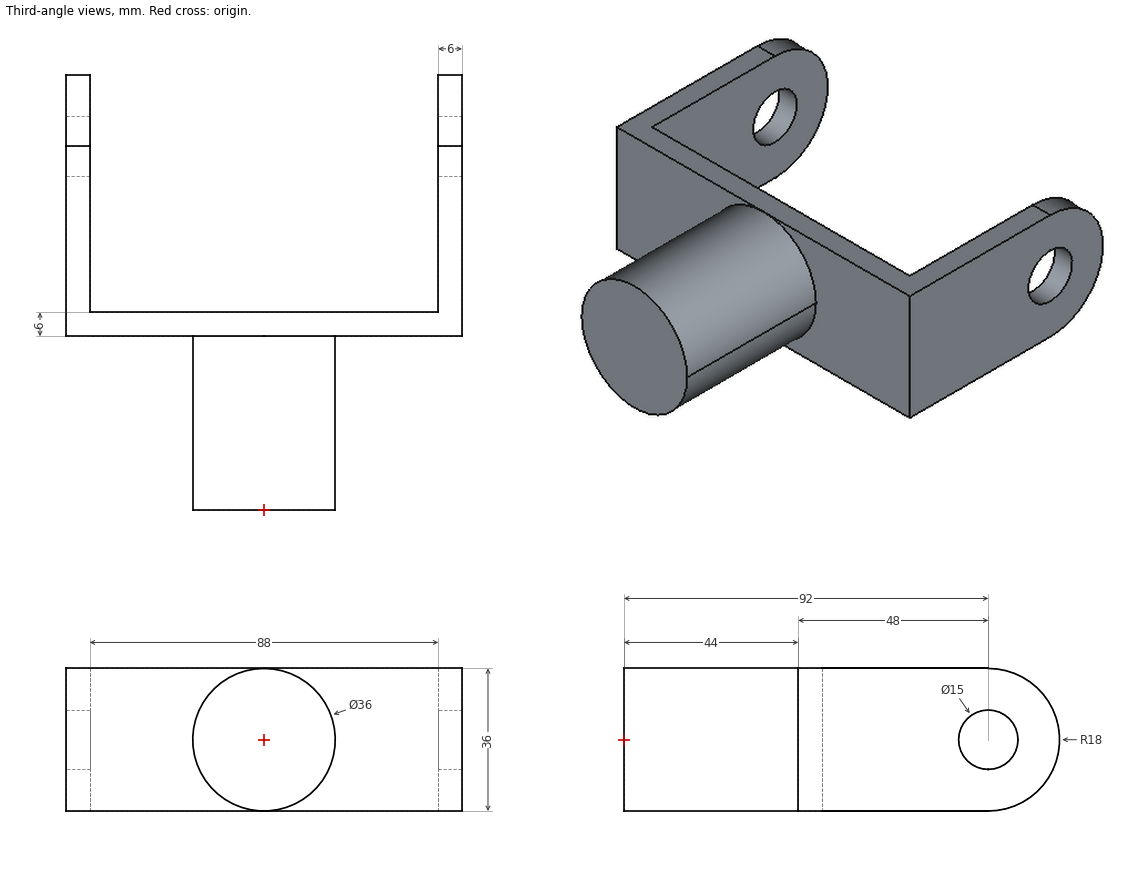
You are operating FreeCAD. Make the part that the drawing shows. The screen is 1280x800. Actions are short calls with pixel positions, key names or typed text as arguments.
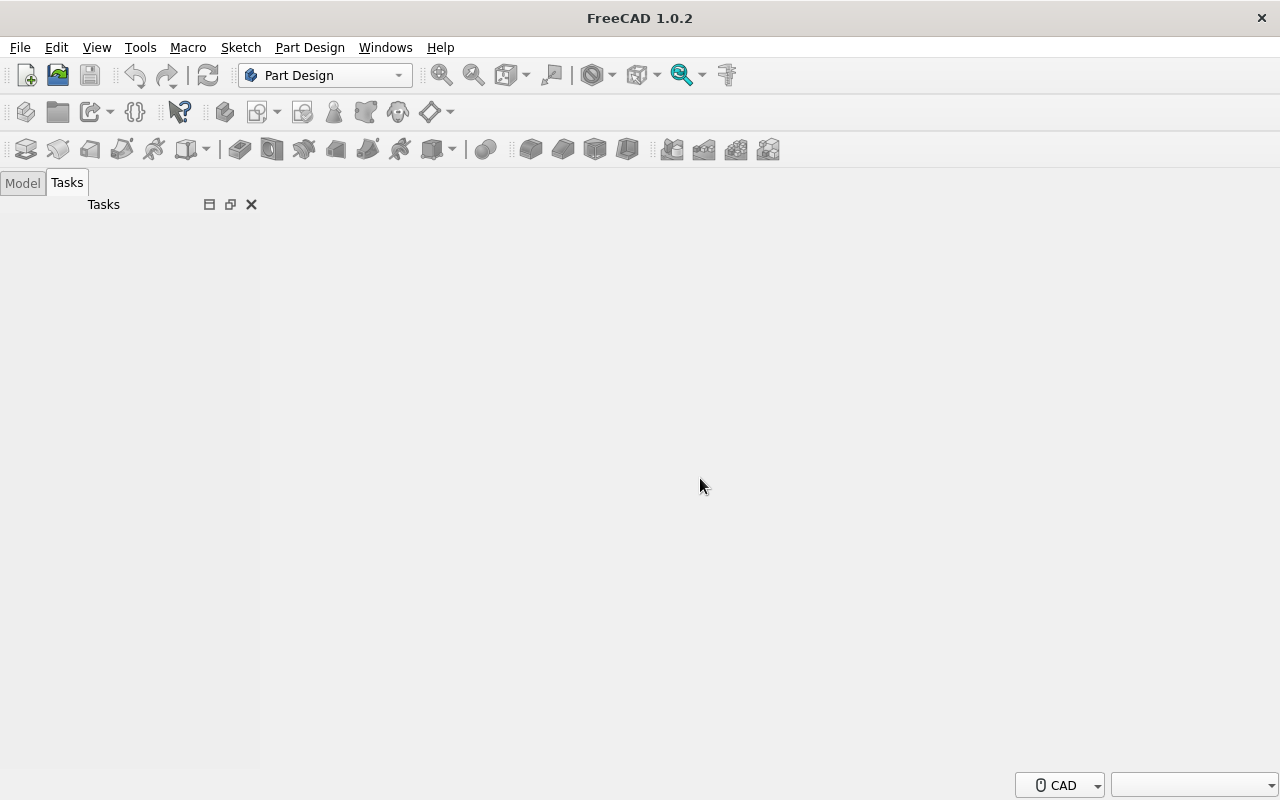
key(ctrl+n)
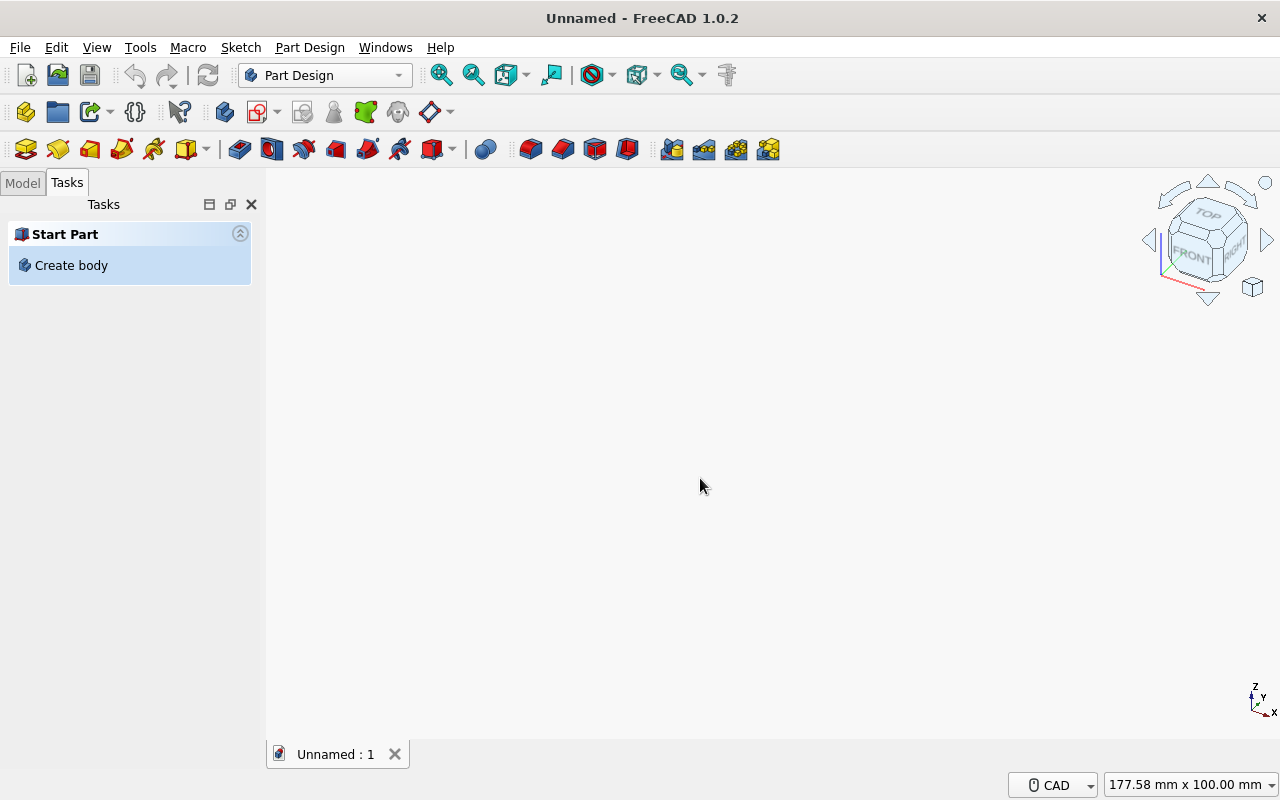
click(258, 112)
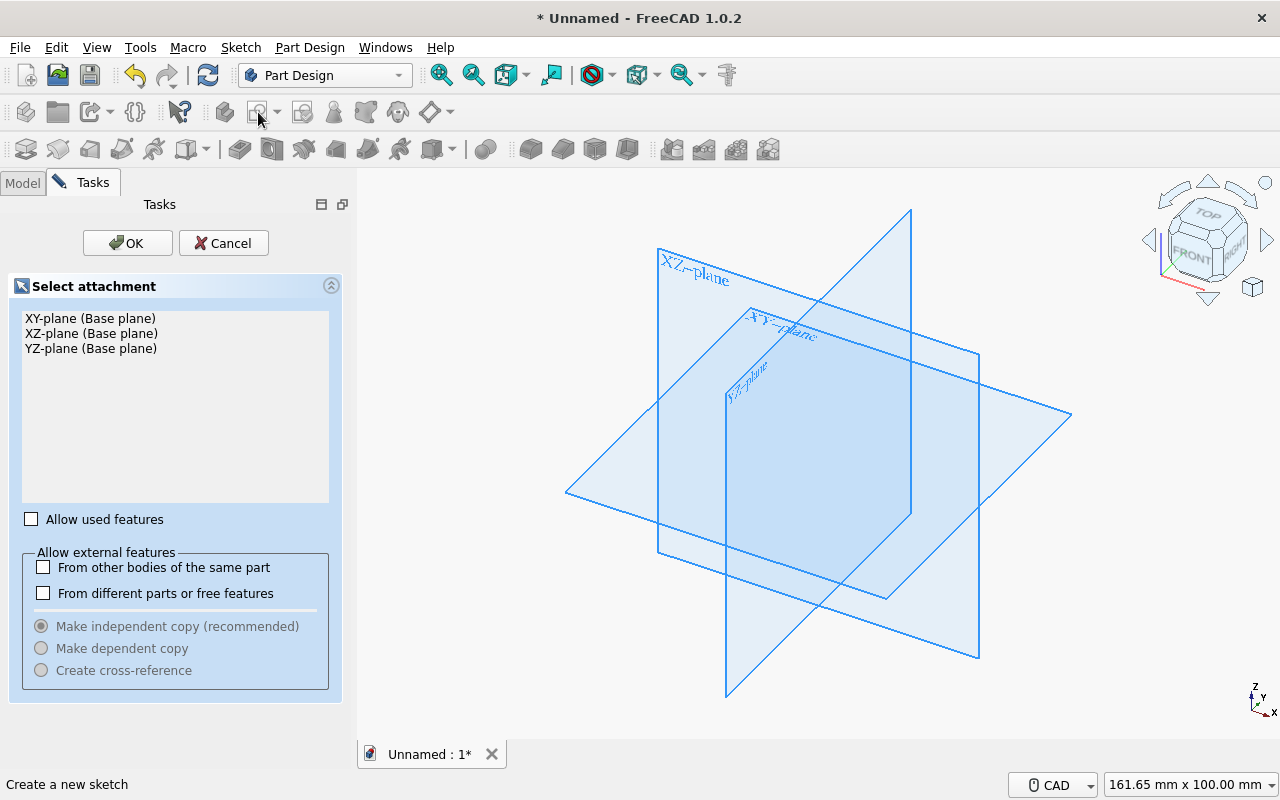
click(82, 334)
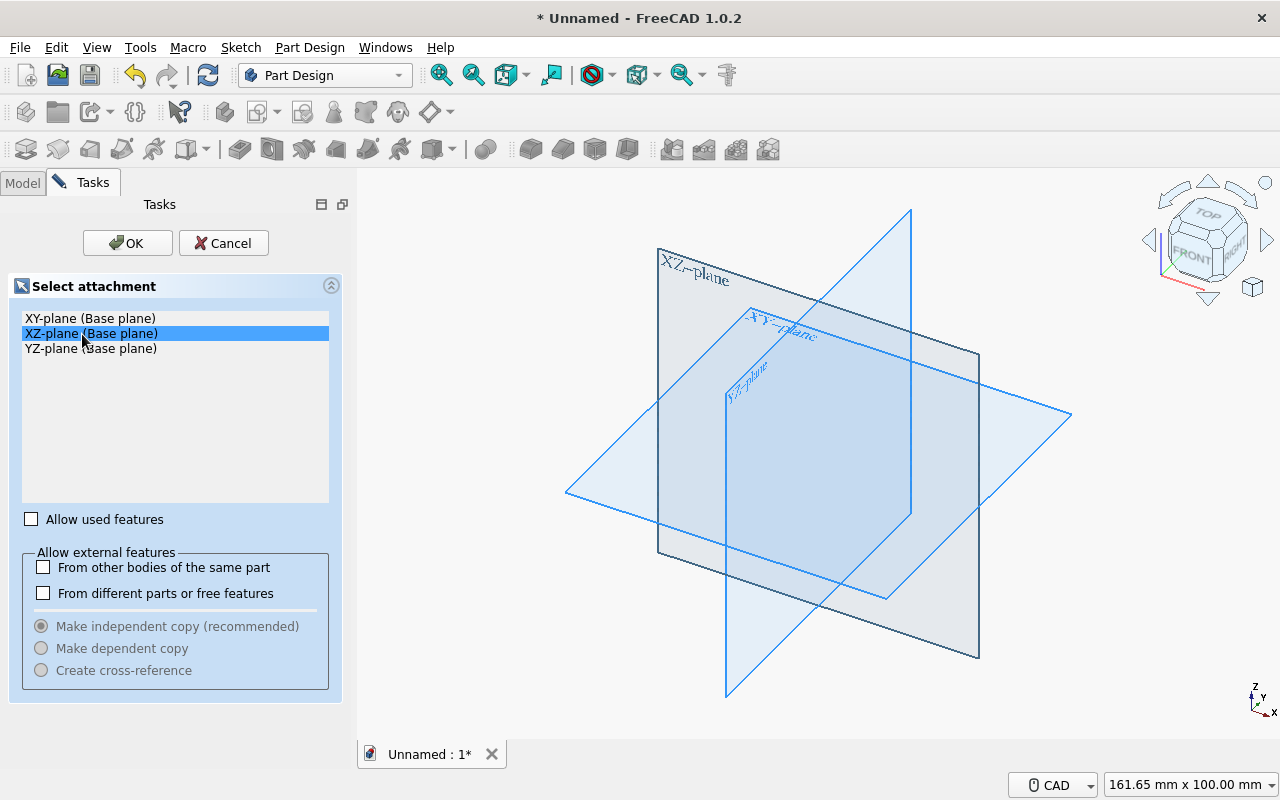
click(128, 243)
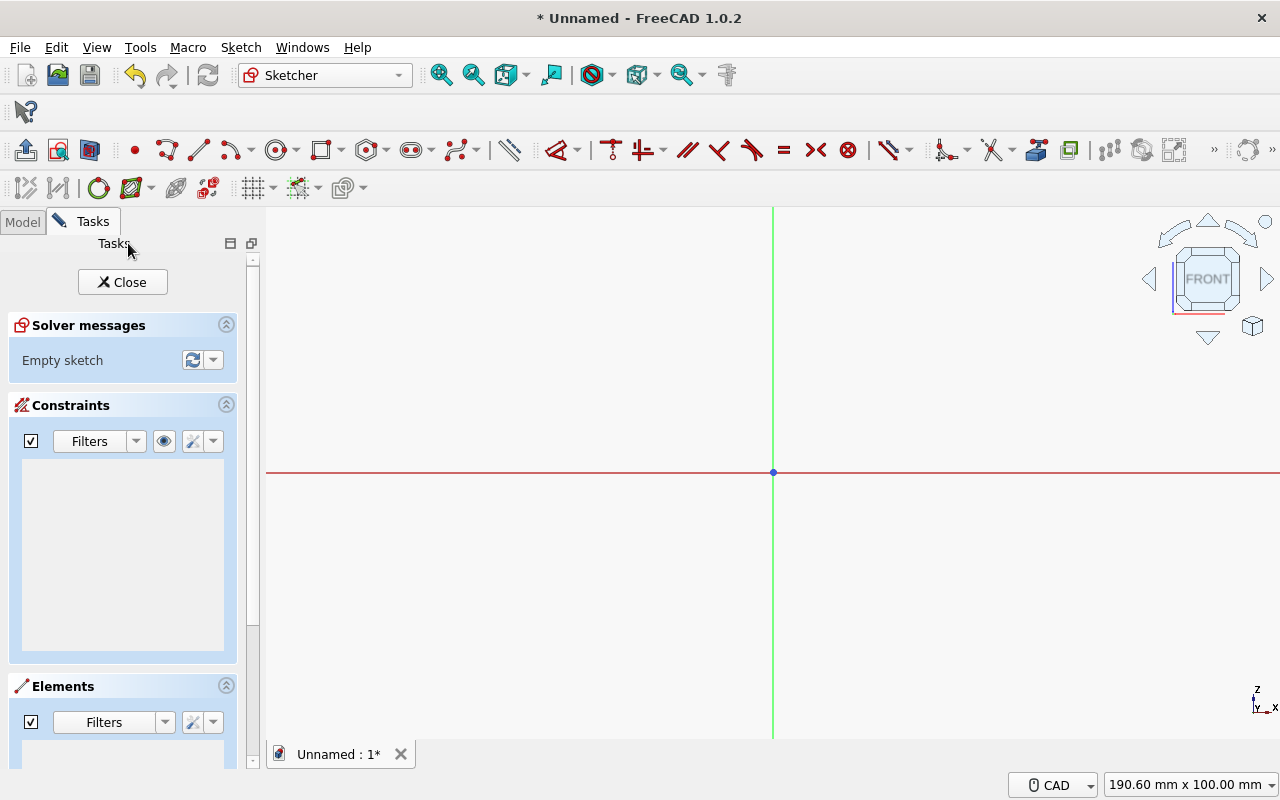
scroll(856, 473, up, 3)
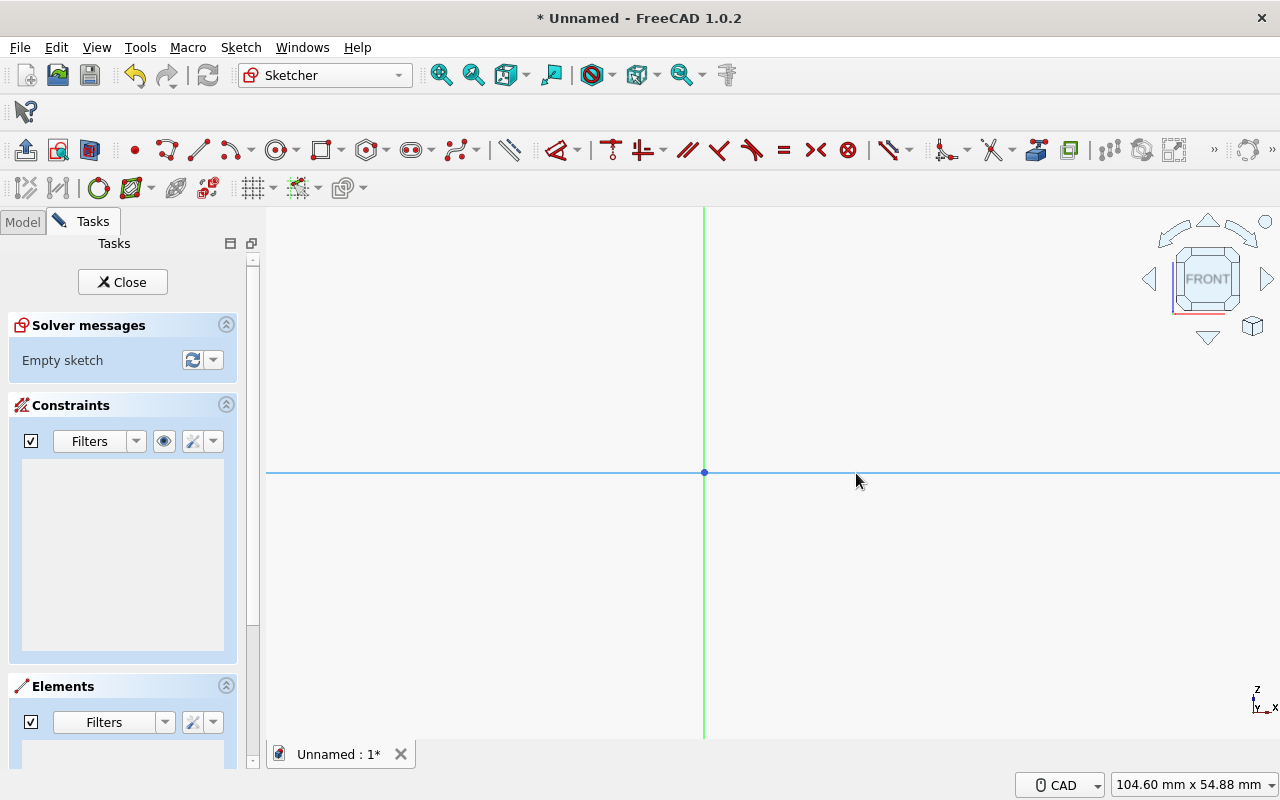
key(g)
key(c)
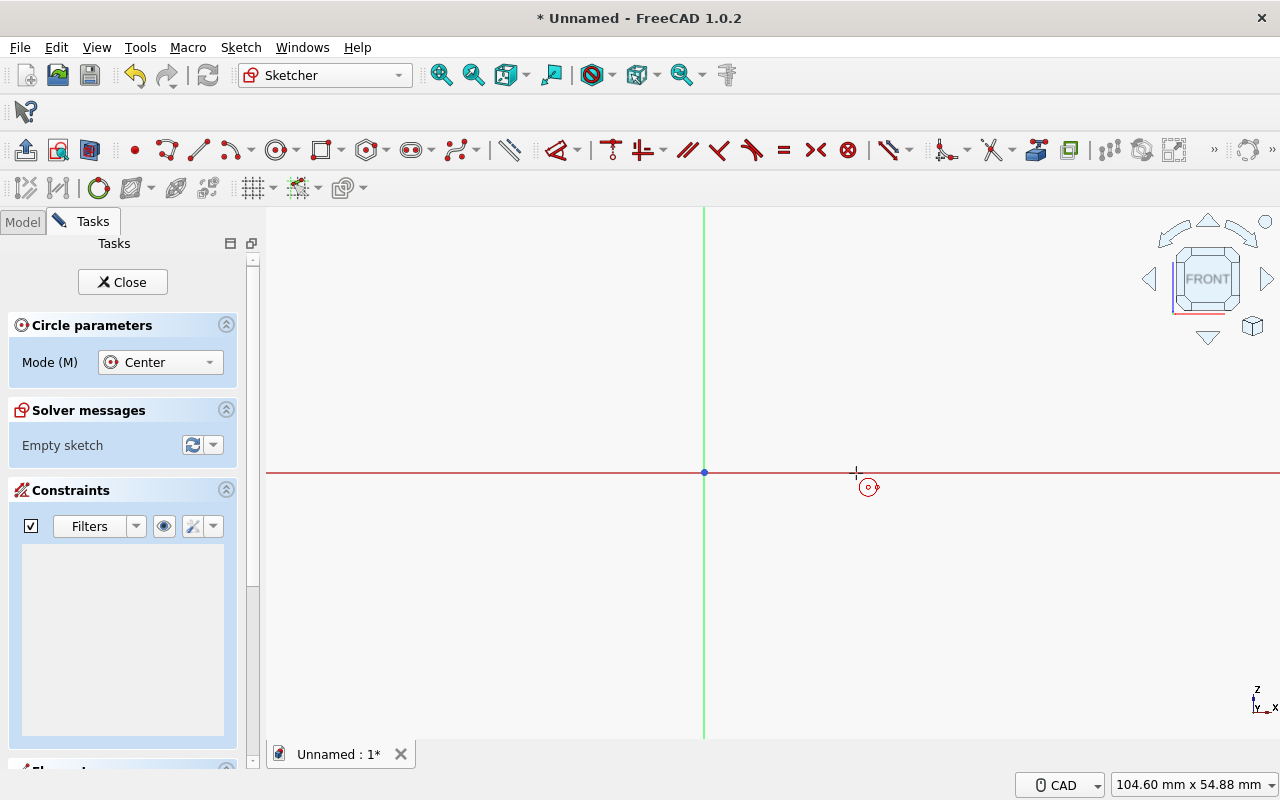
click(704, 473)
click(828, 349)
key(Escape)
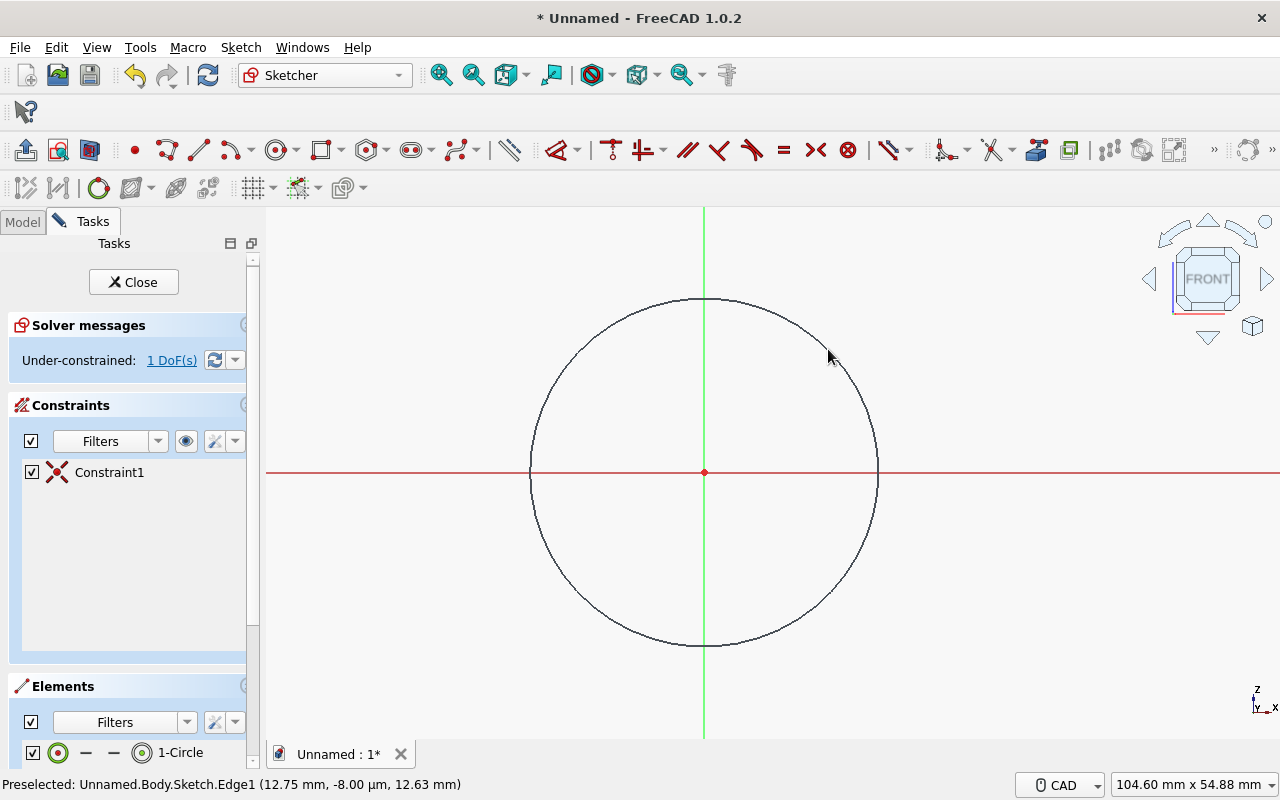
click(827, 349)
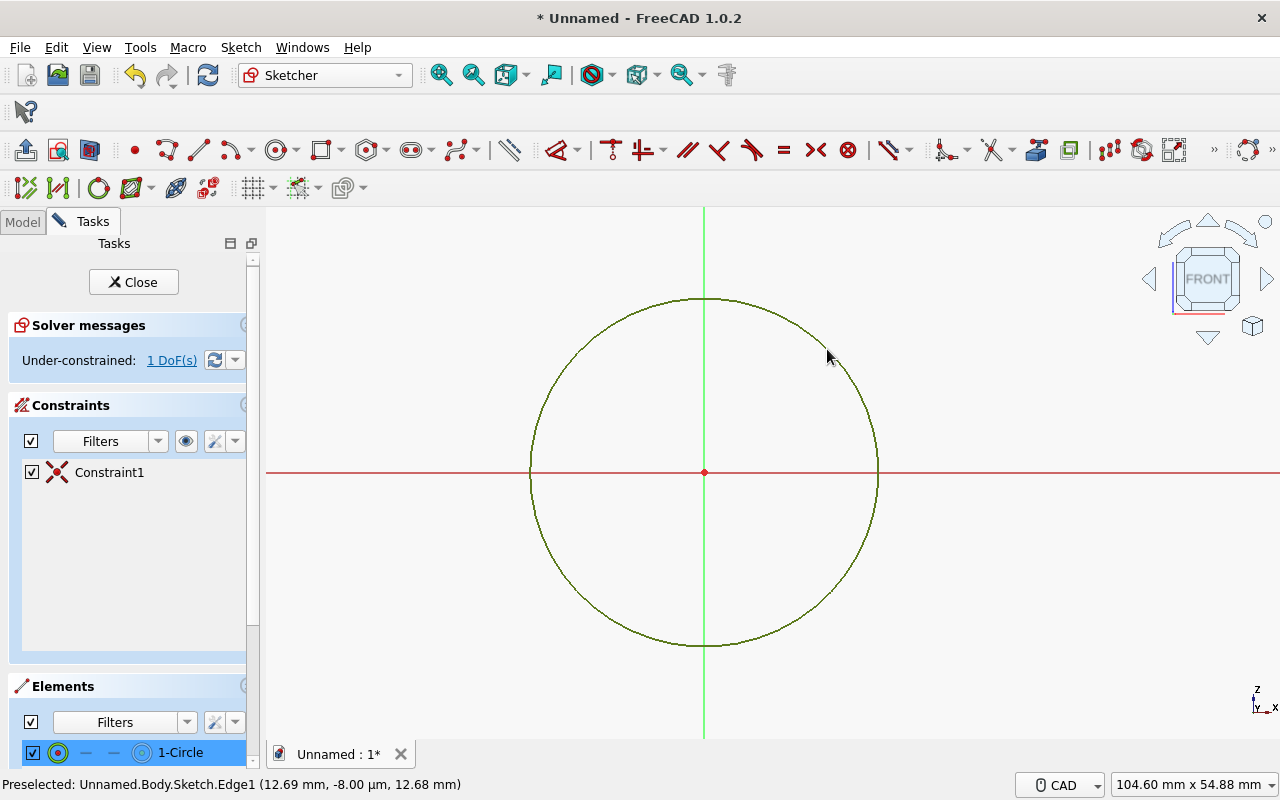
key(k)
key(o)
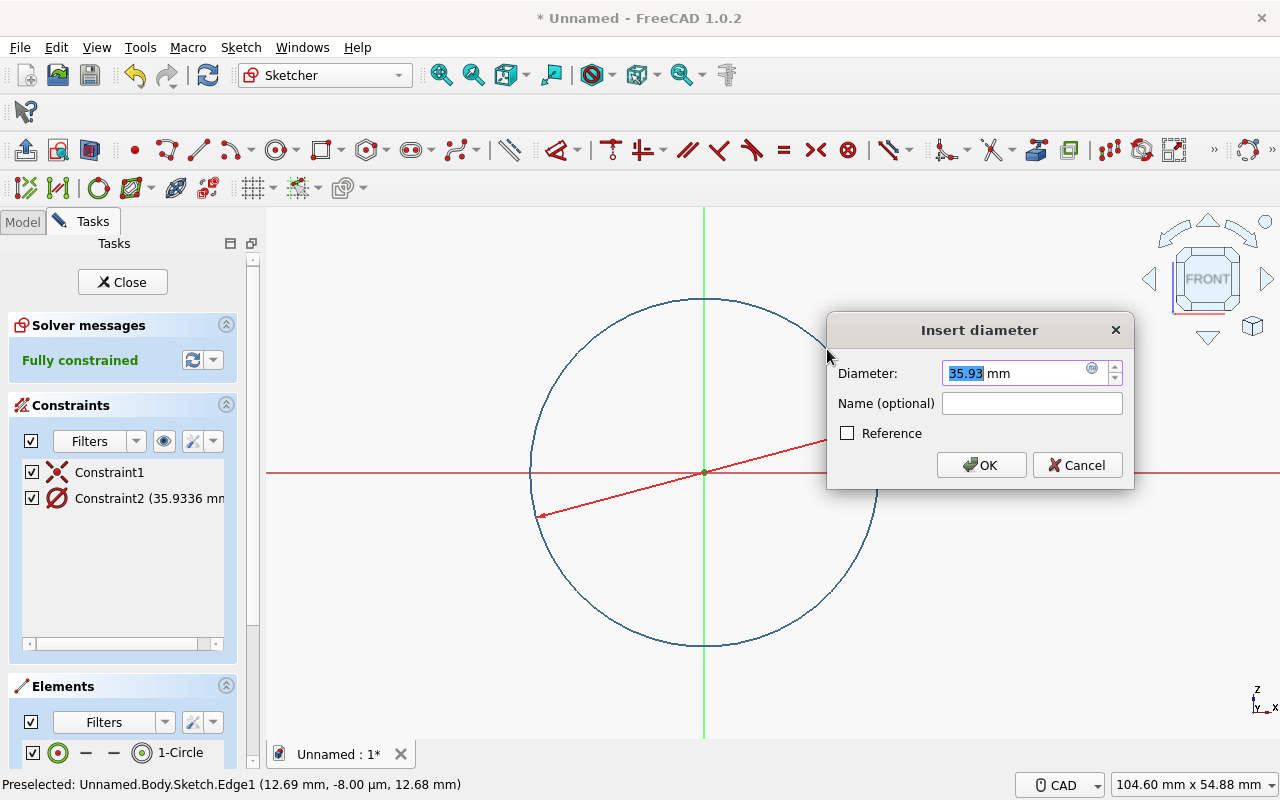
text(36)
key(Return)